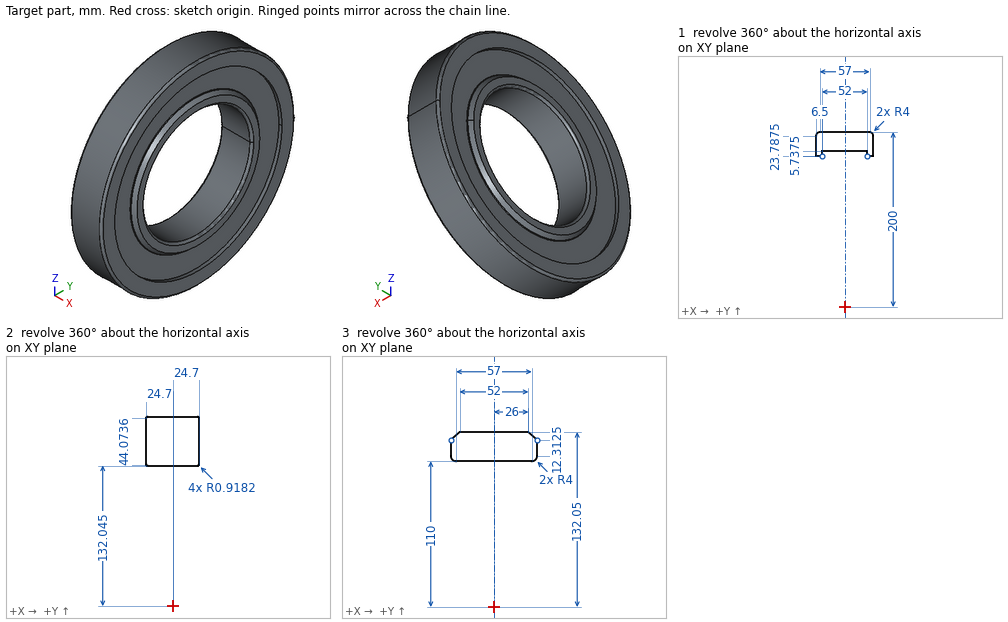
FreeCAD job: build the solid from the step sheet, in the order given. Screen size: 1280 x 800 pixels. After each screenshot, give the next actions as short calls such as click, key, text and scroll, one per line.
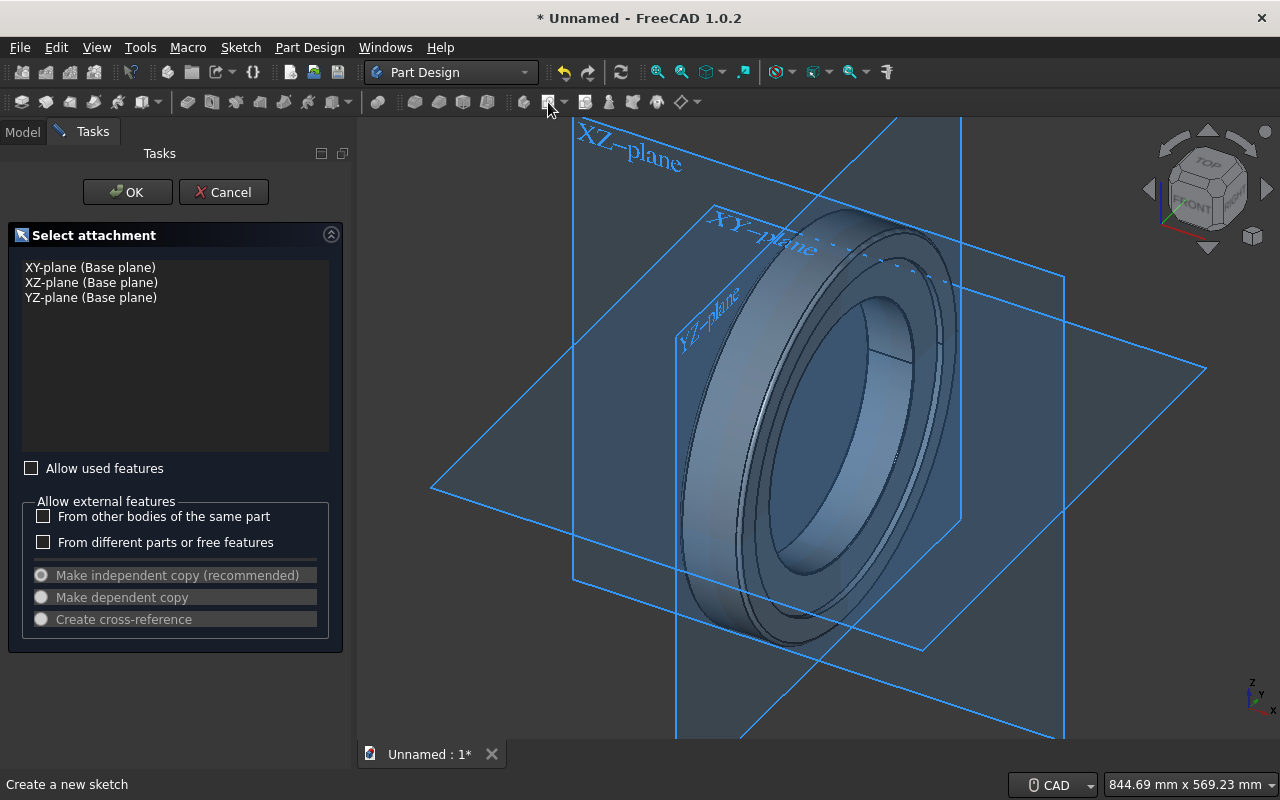
click(82, 268)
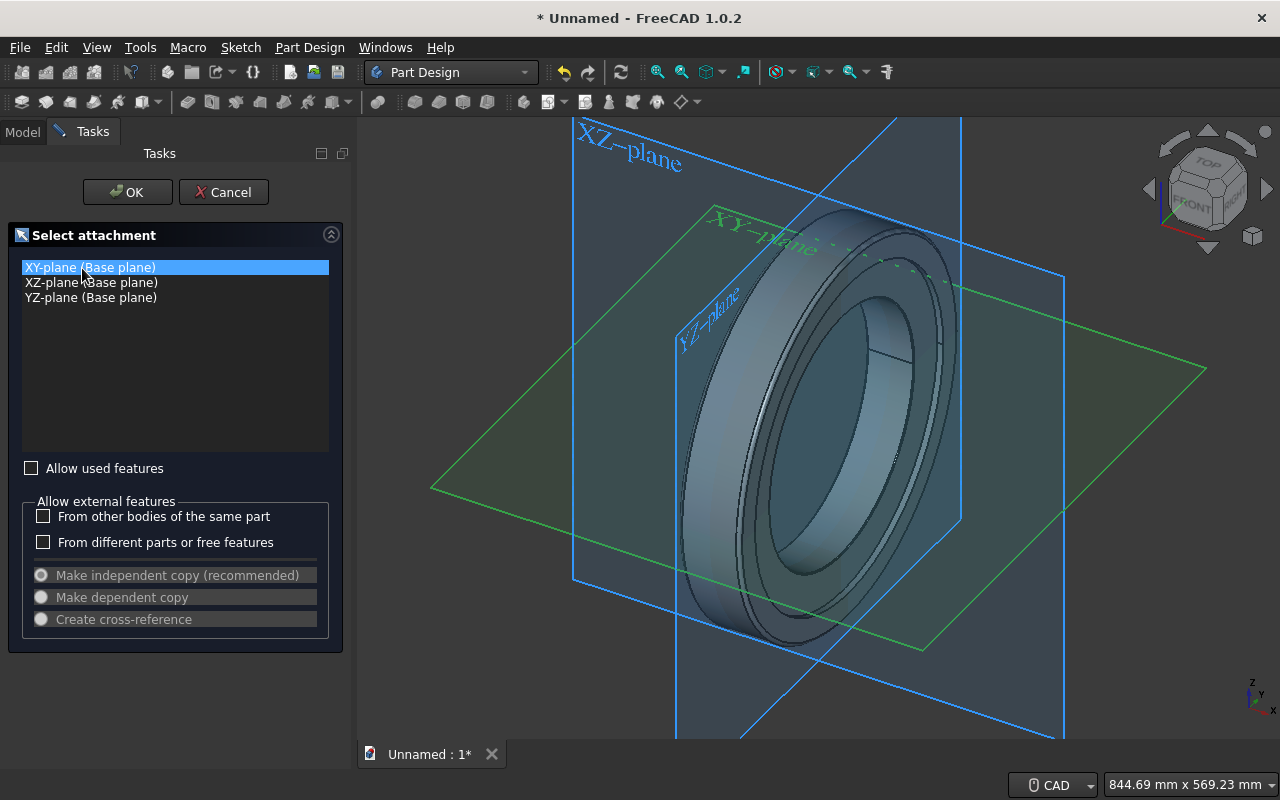
click(128, 192)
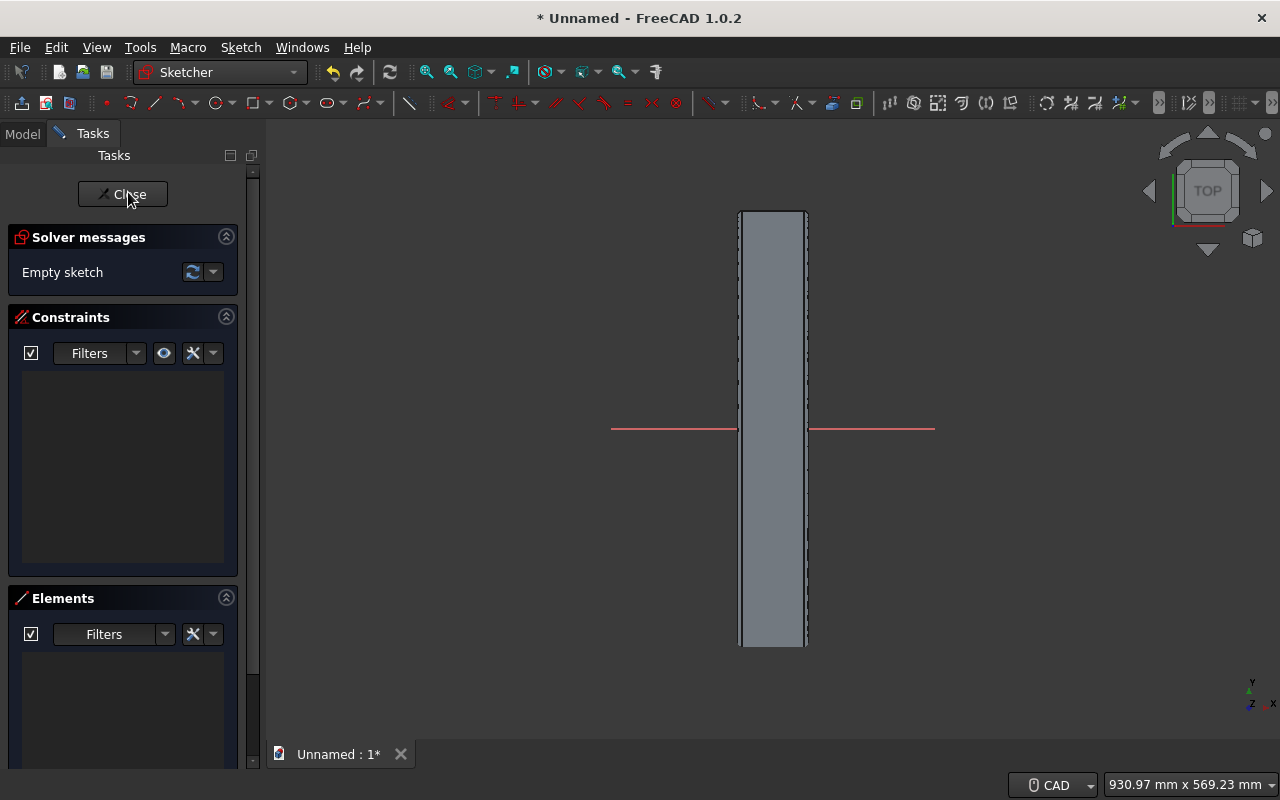
click(70, 104)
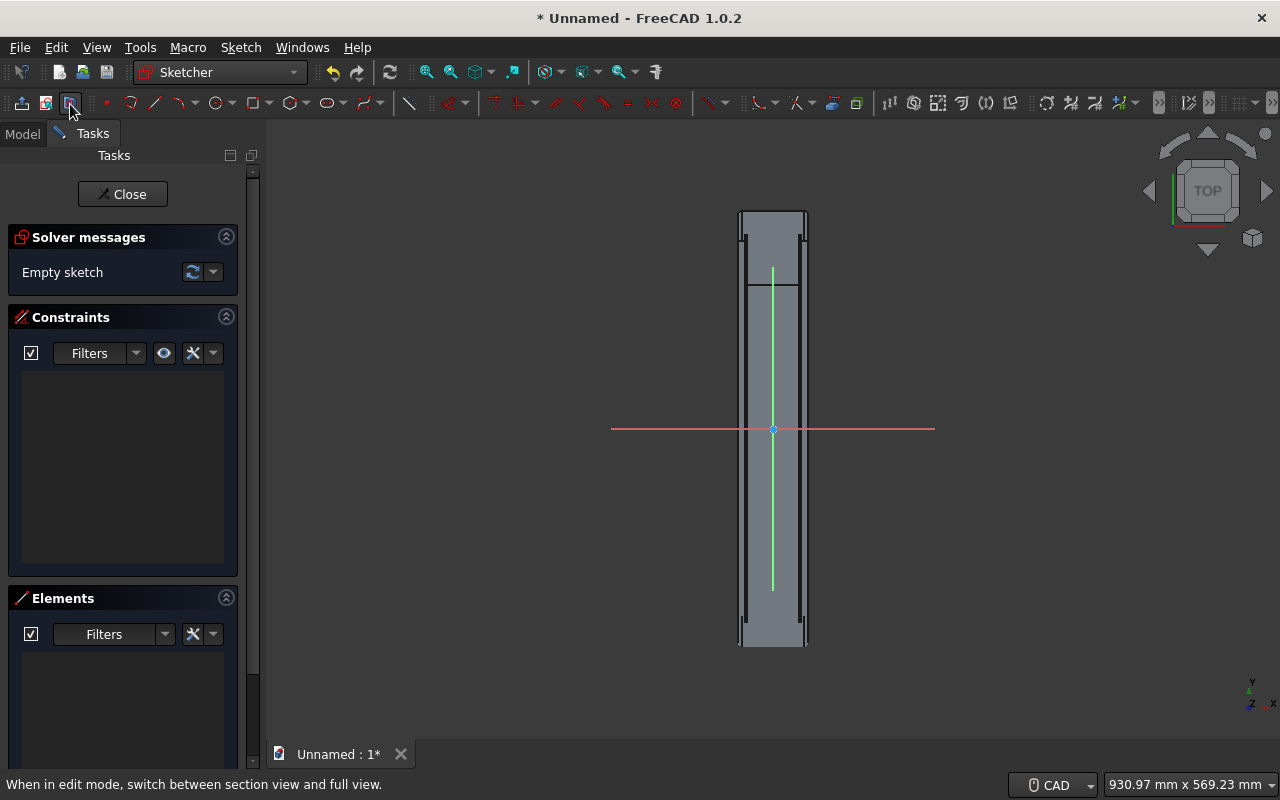
scroll(813, 315, up, 5)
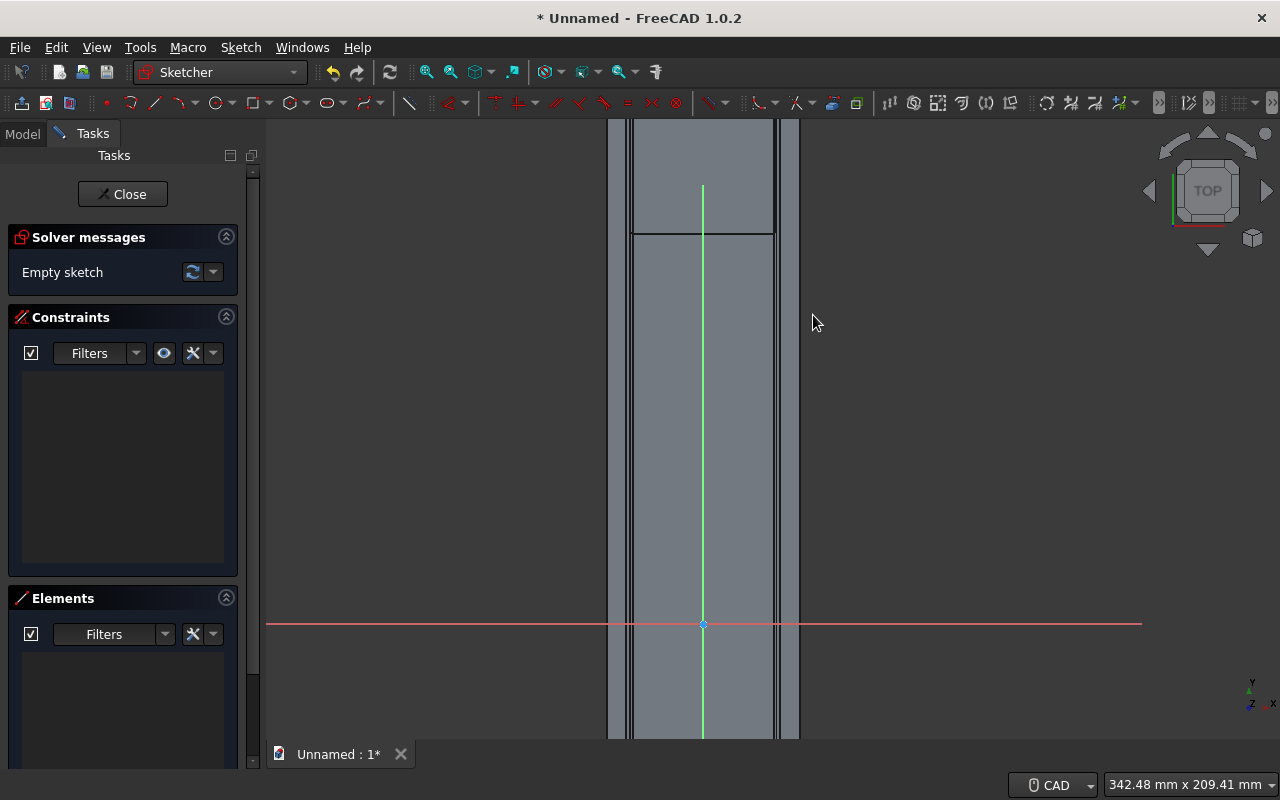
click(156, 104)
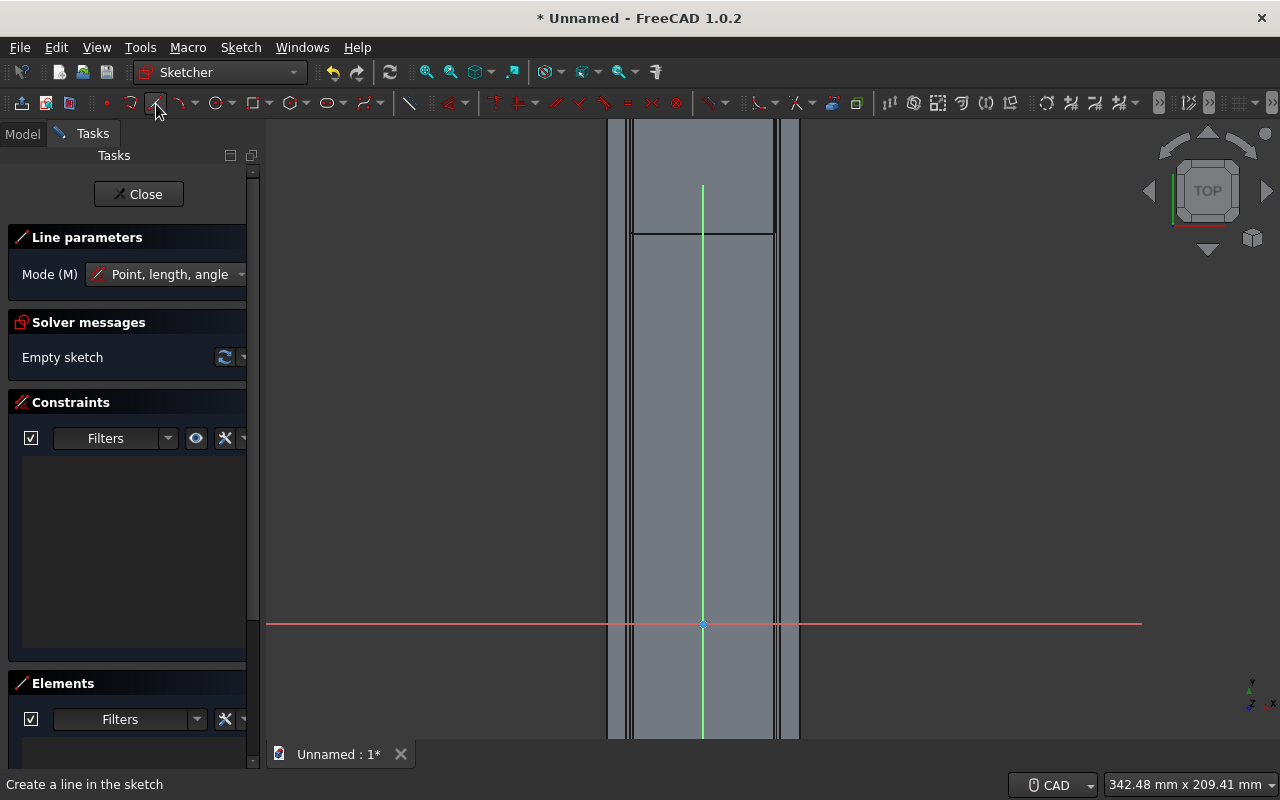
click(619, 299)
click(788, 299)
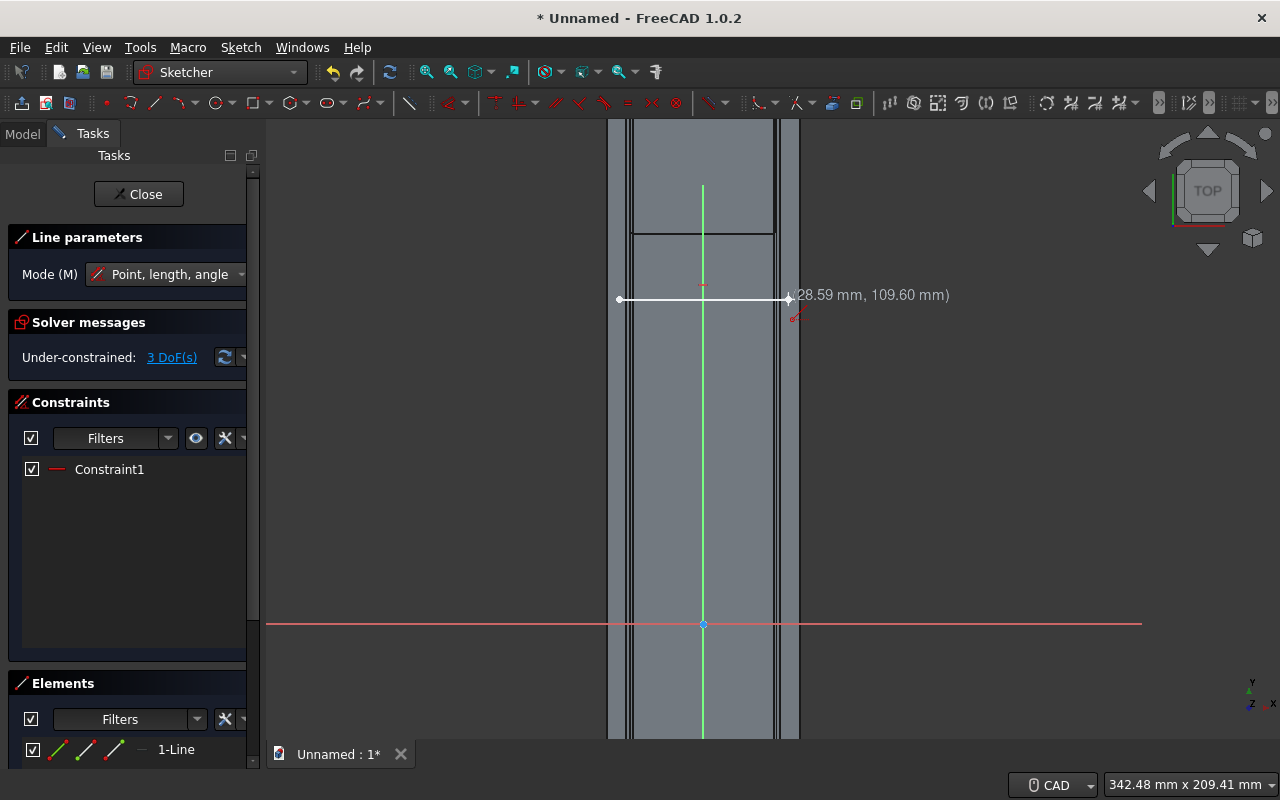
click(132, 104)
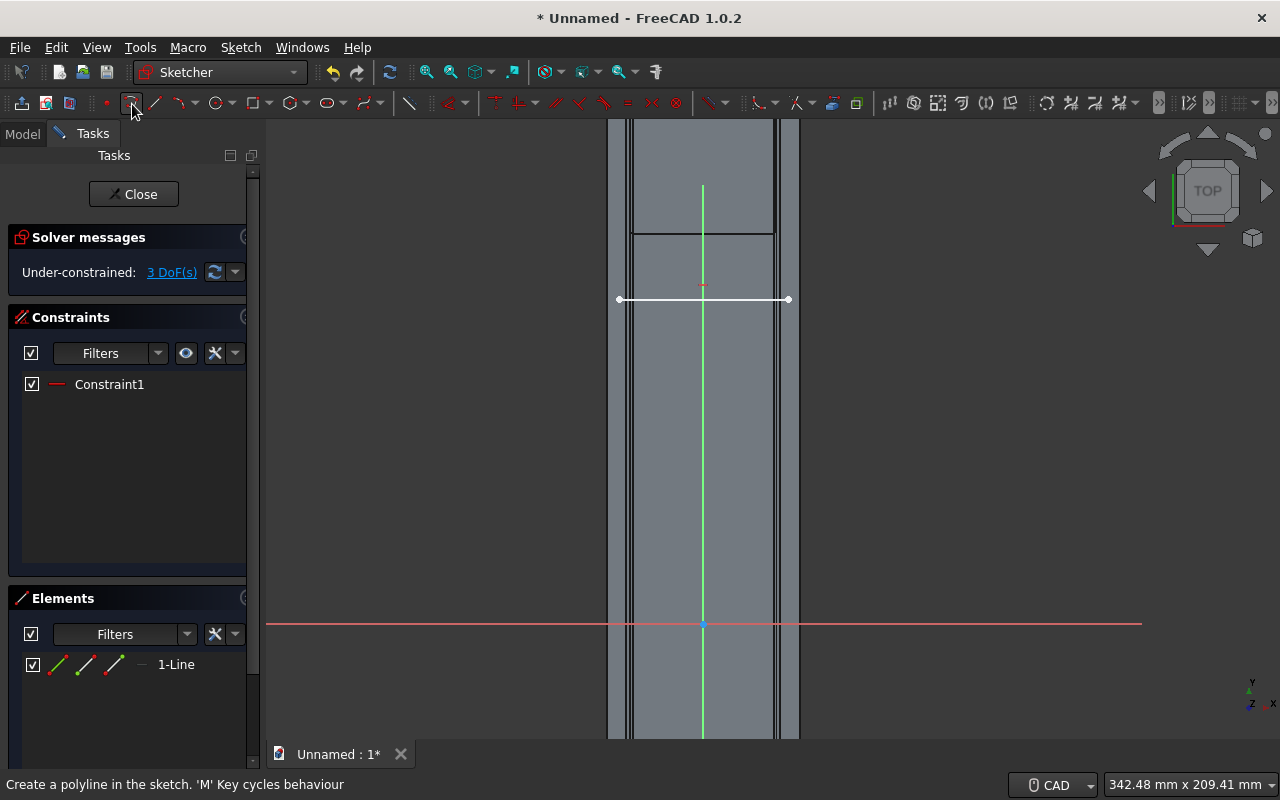
click(800, 287)
click(800, 251)
click(780, 234)
click(626, 234)
click(607, 251)
click(607, 287)
right_click(607, 287)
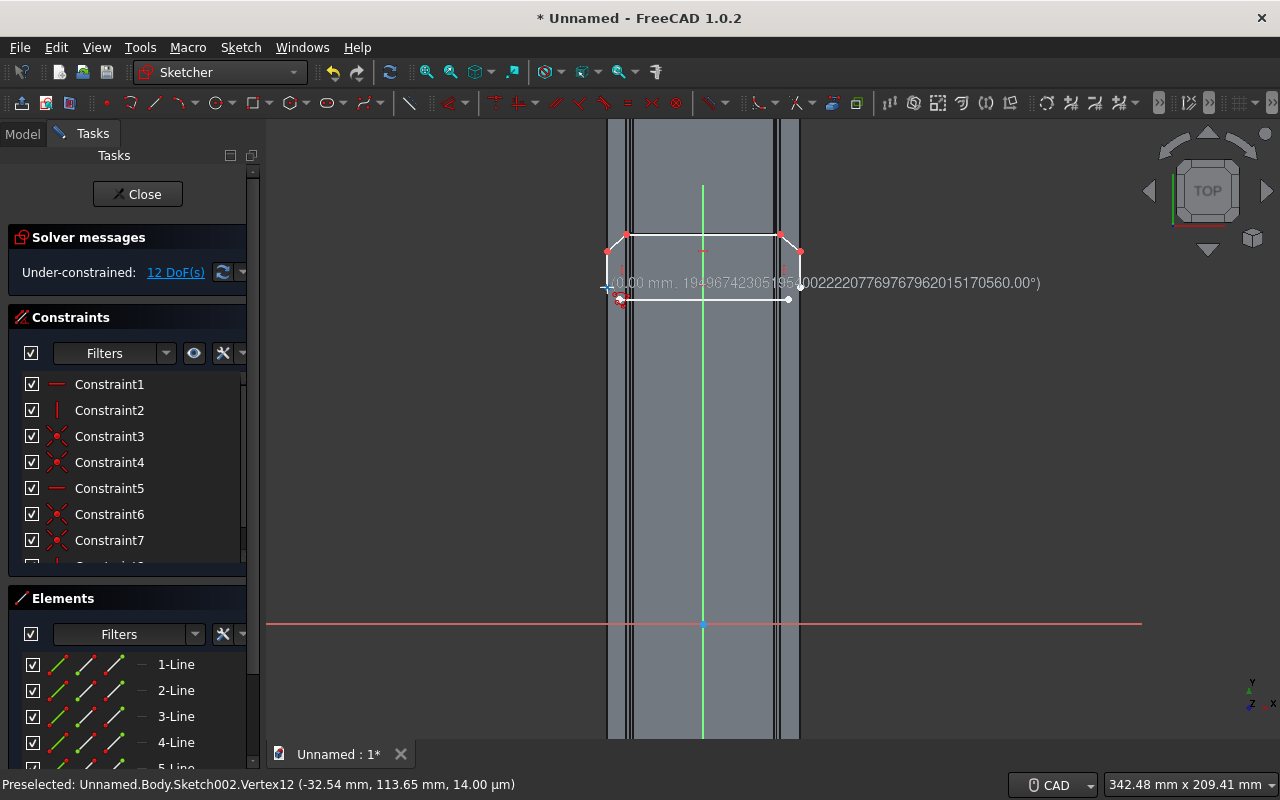
click(180, 104)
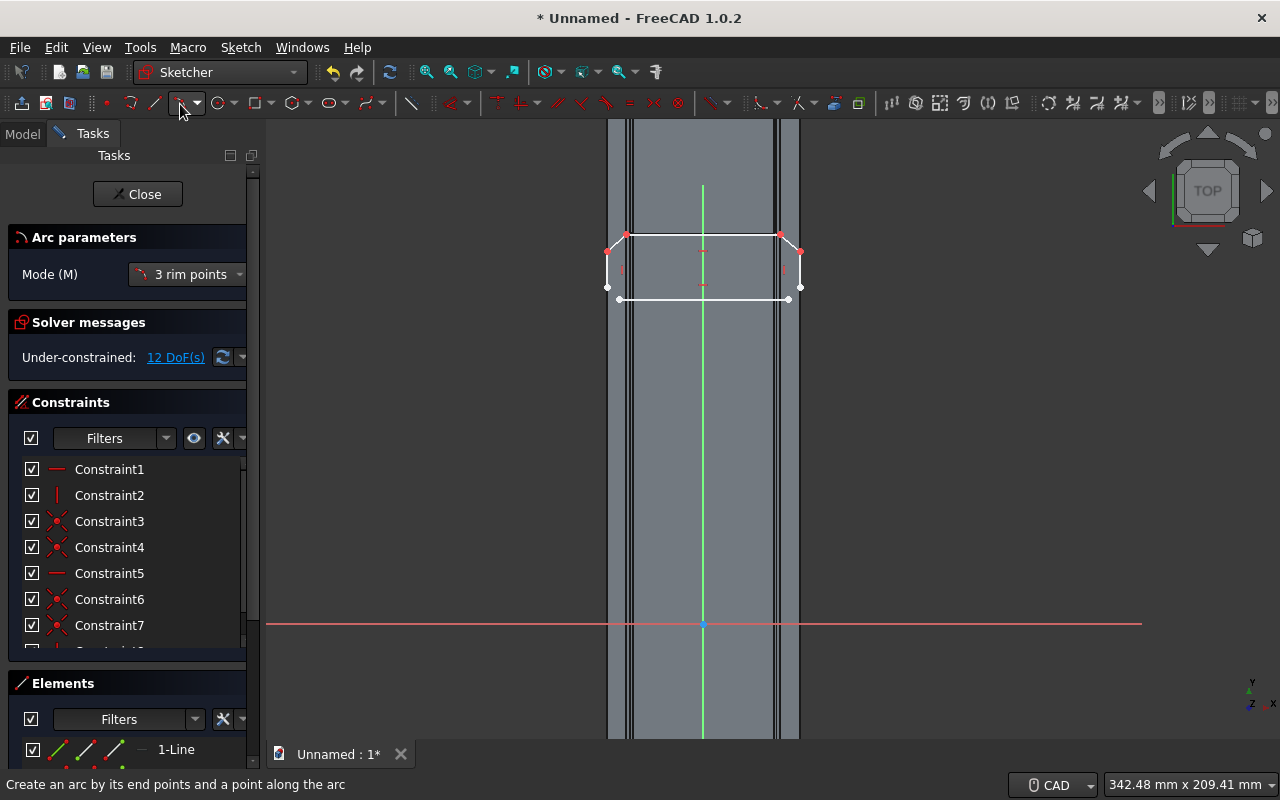
click(788, 300)
click(800, 288)